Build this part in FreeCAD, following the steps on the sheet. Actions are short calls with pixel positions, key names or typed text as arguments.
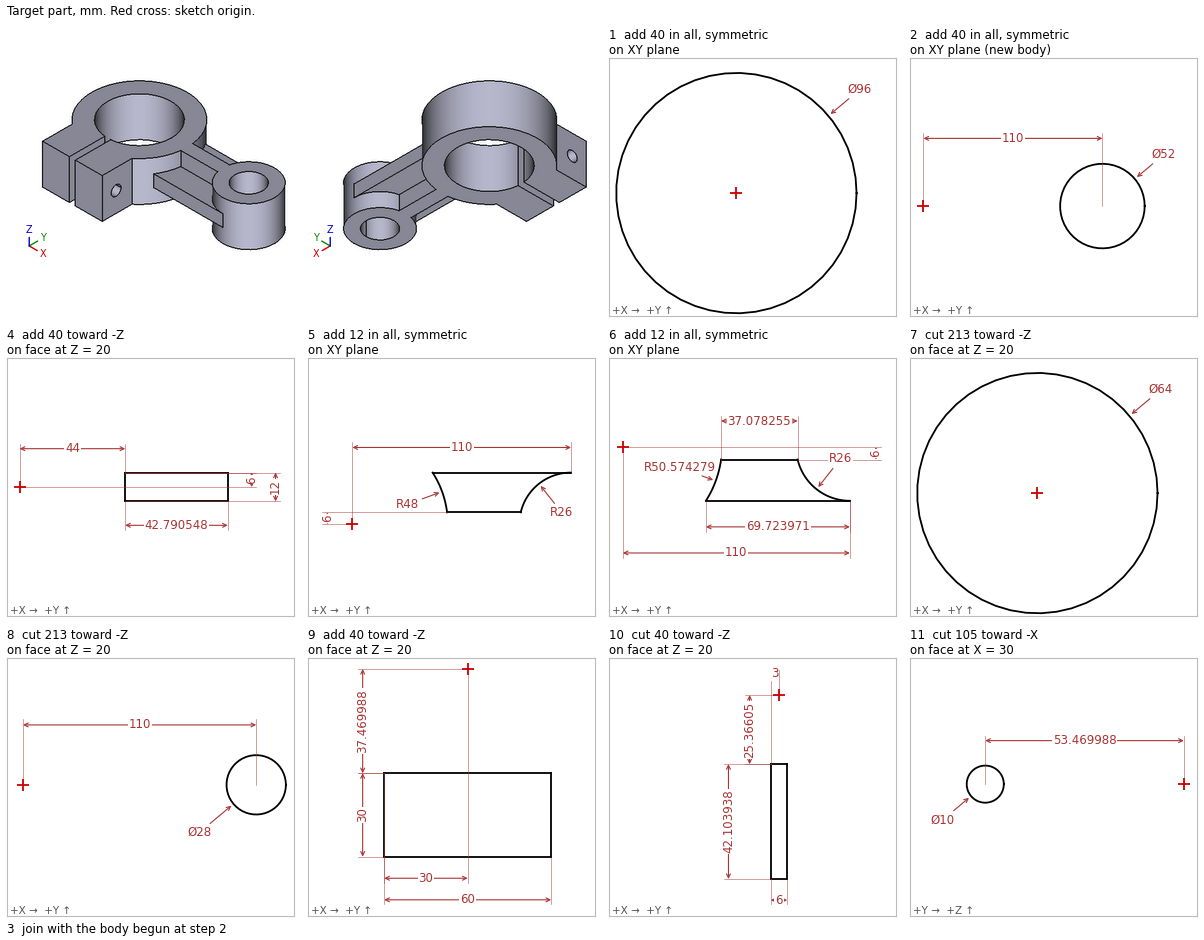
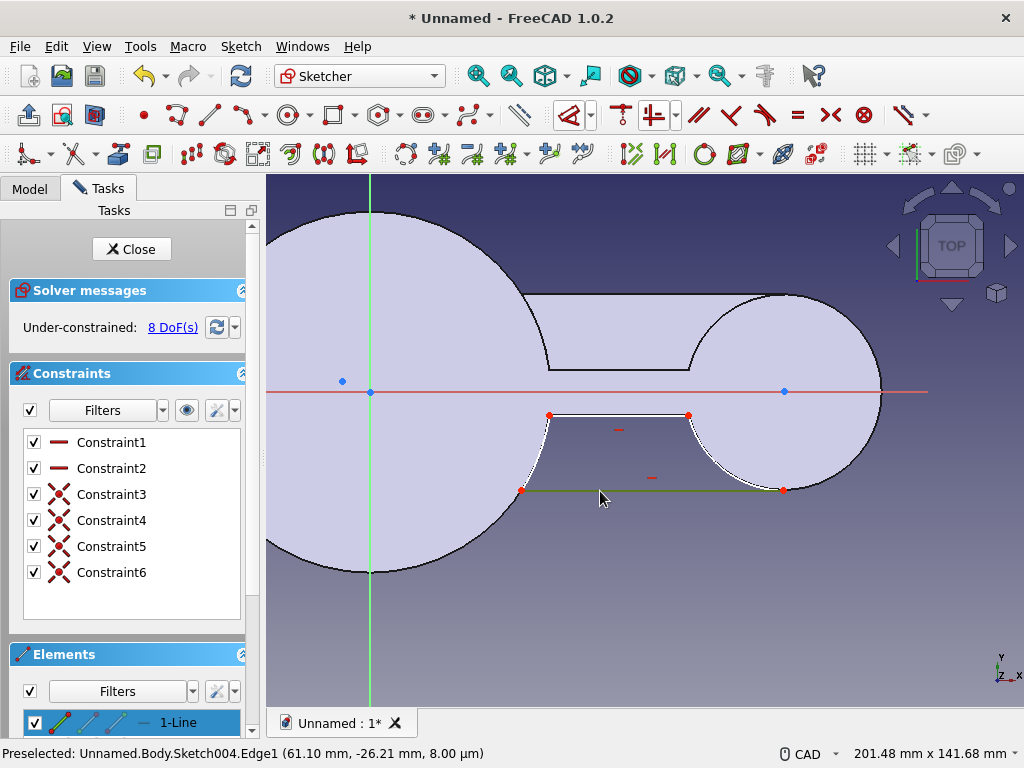
click(705, 451)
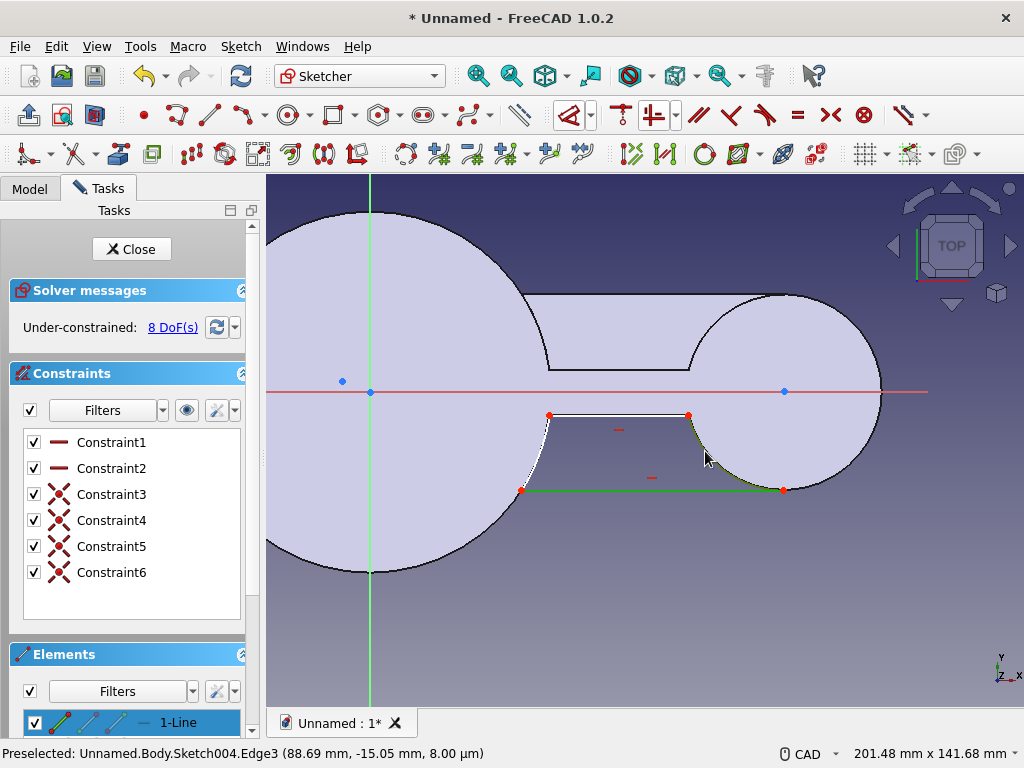
click(765, 116)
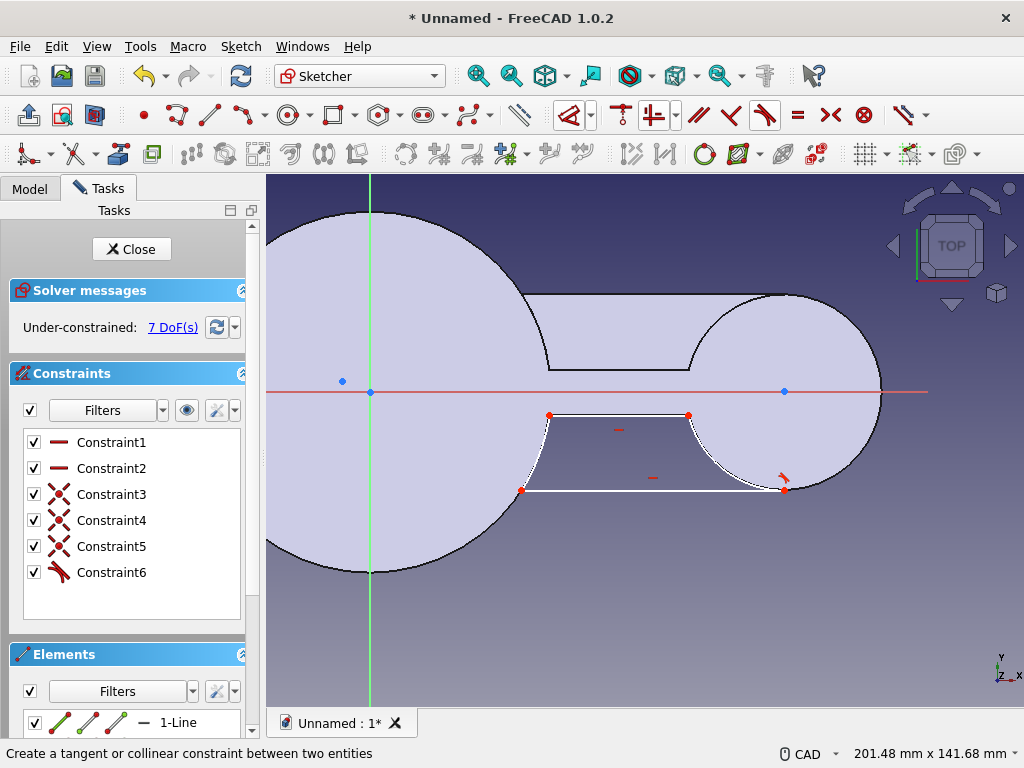
click(785, 392)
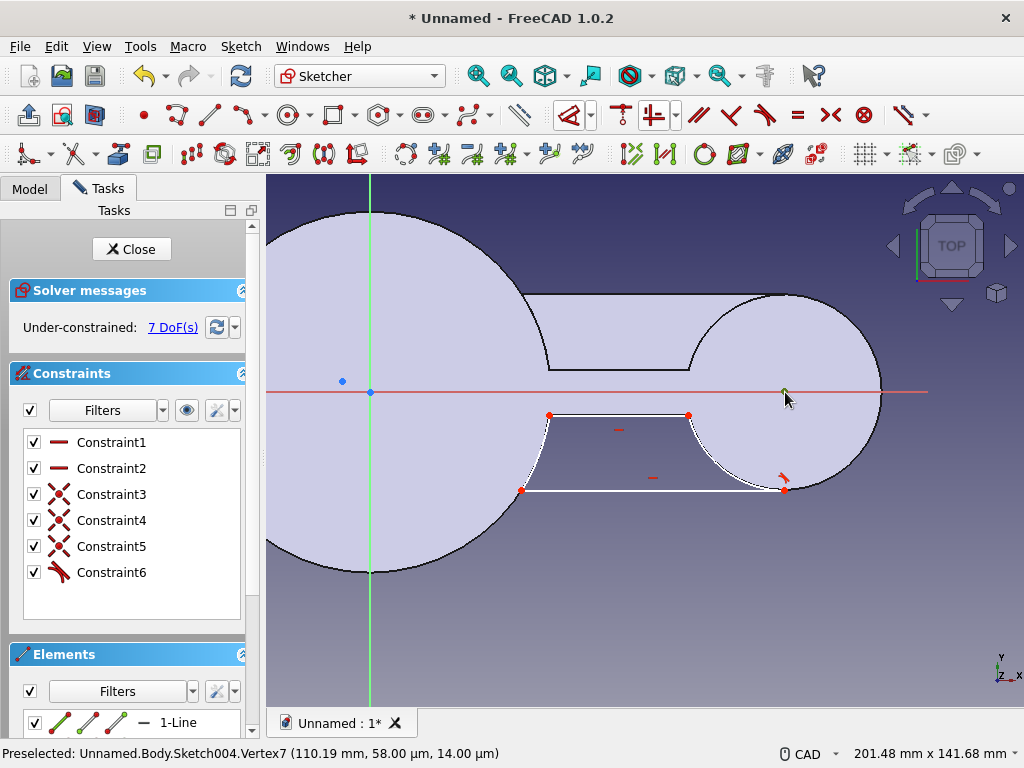
click(334, 392)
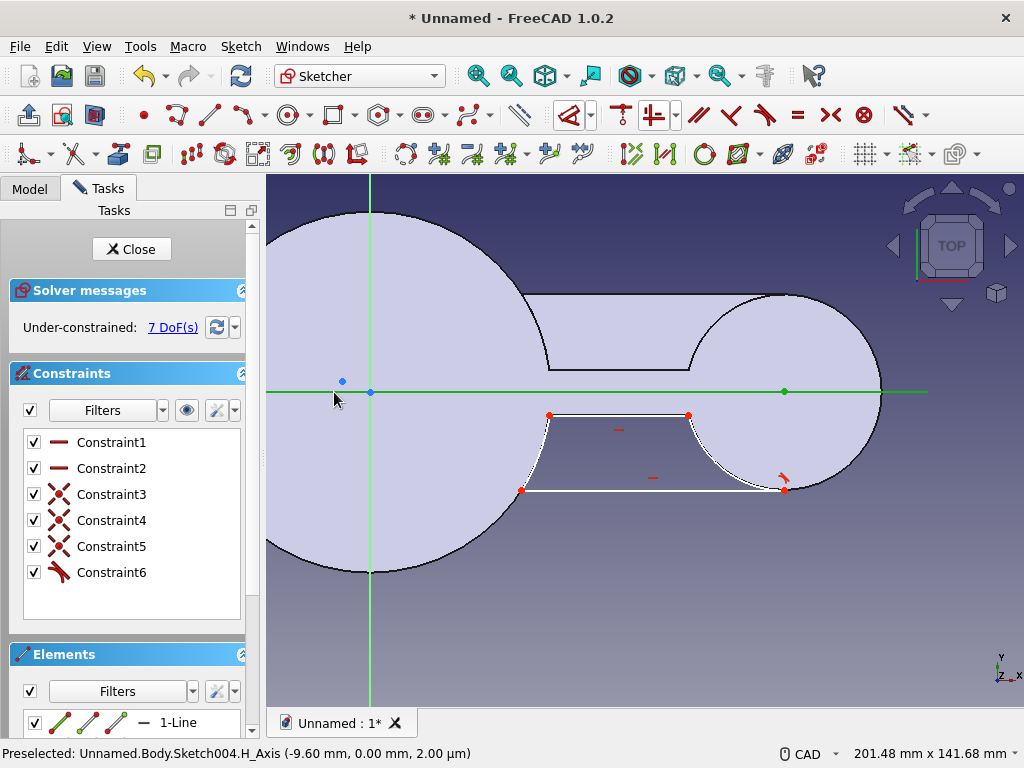
click(621, 116)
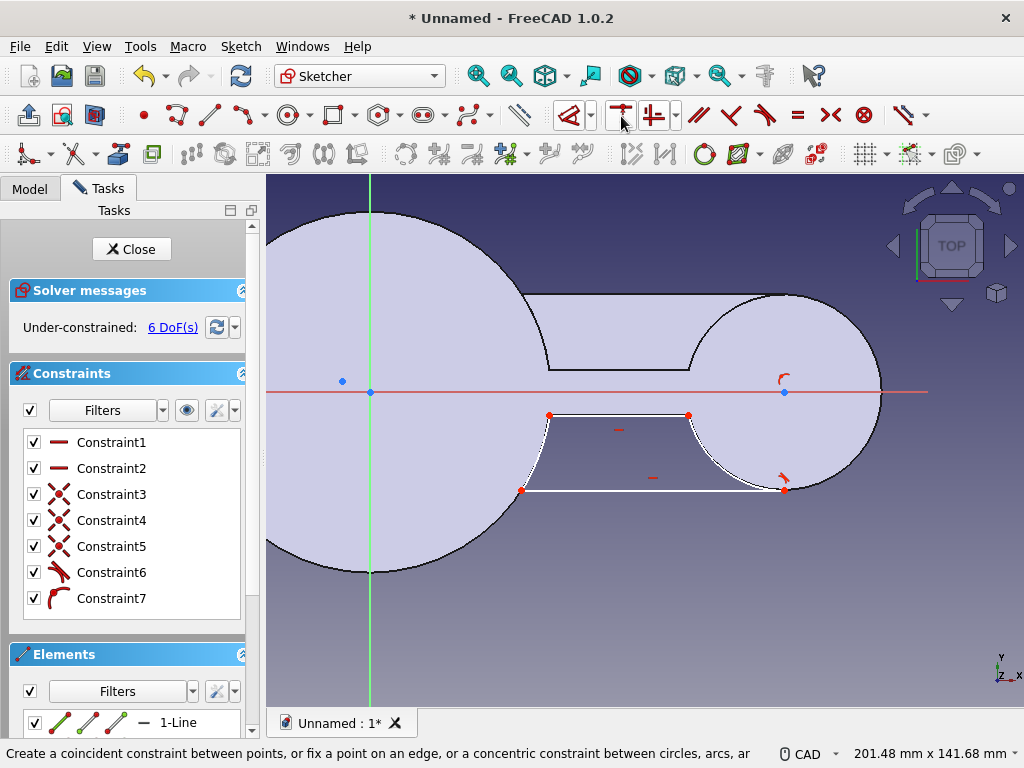
click(705, 451)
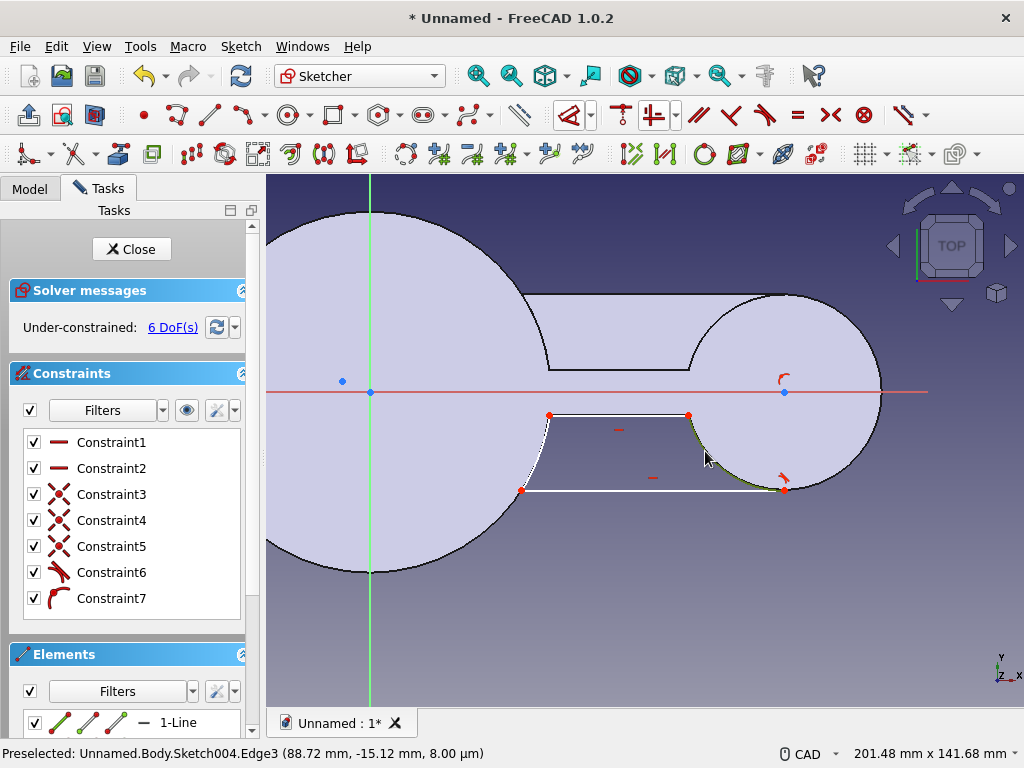
click(590, 116)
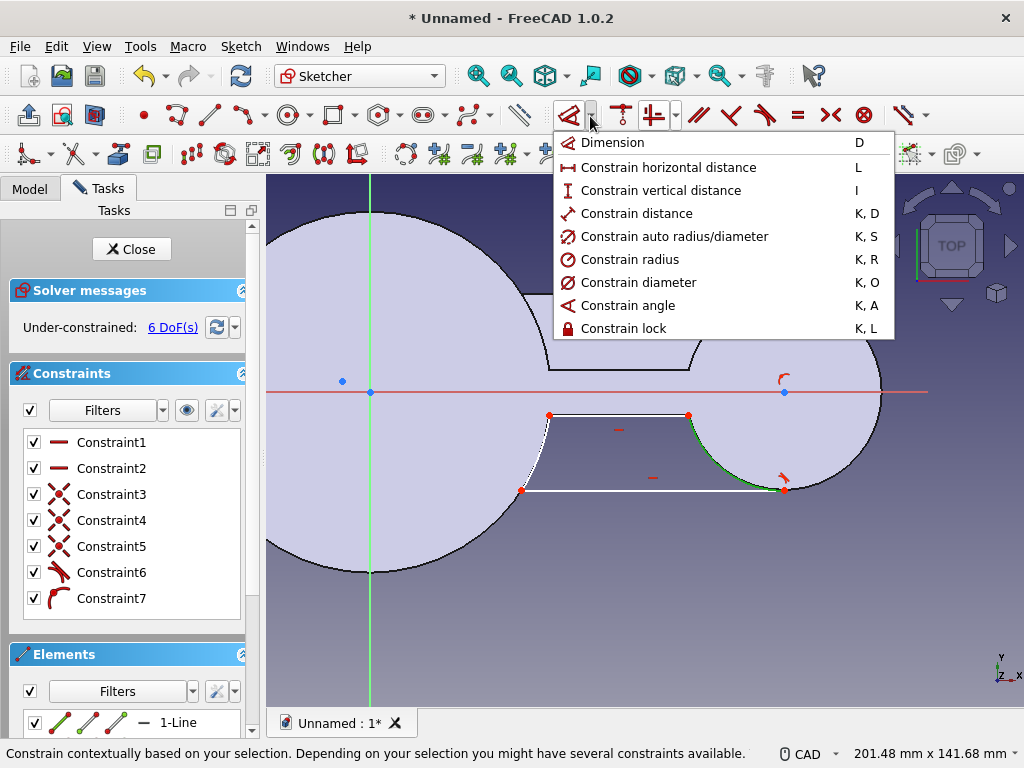
click(724, 260)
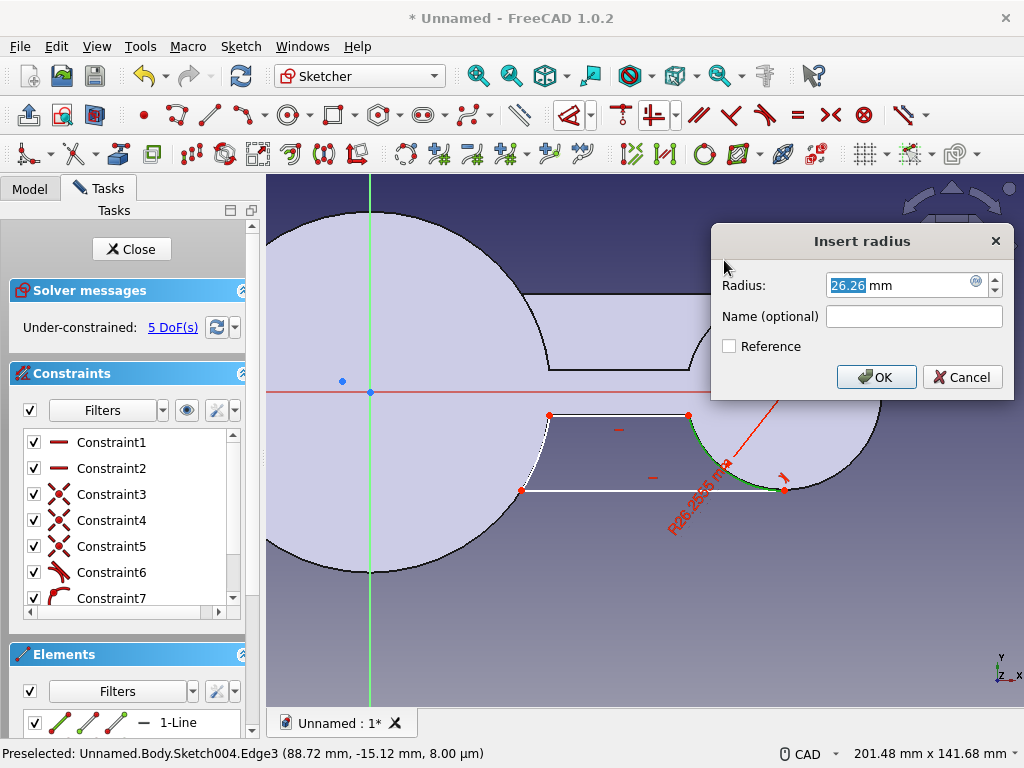
text(26)
key(Return)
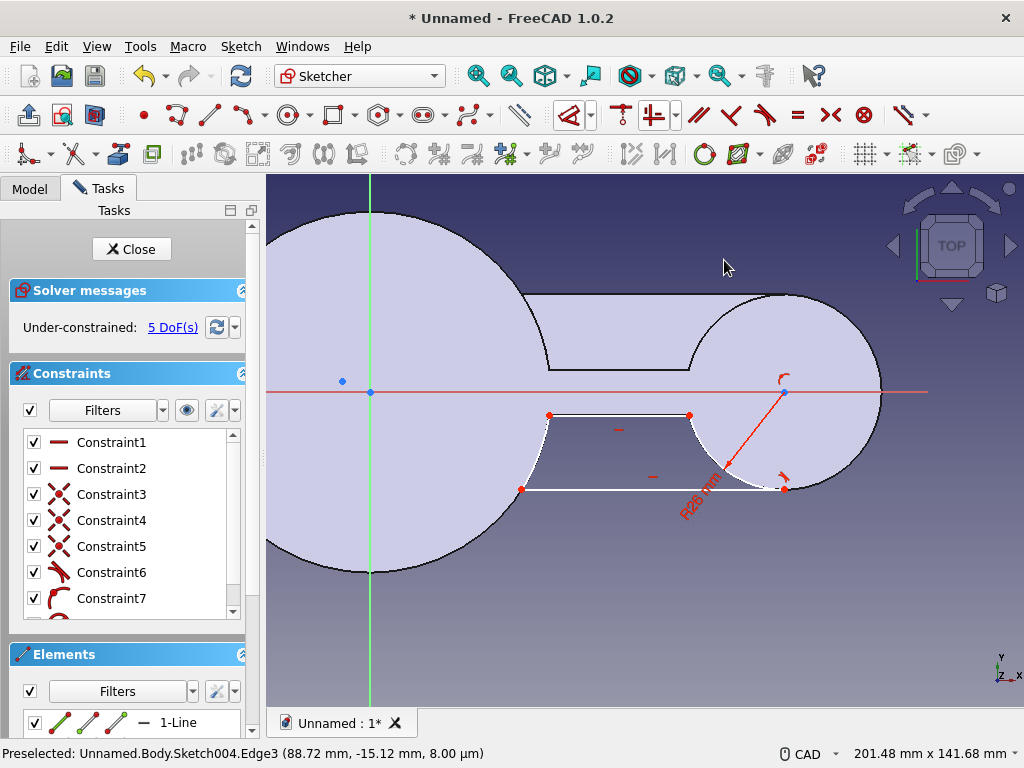
click(533, 469)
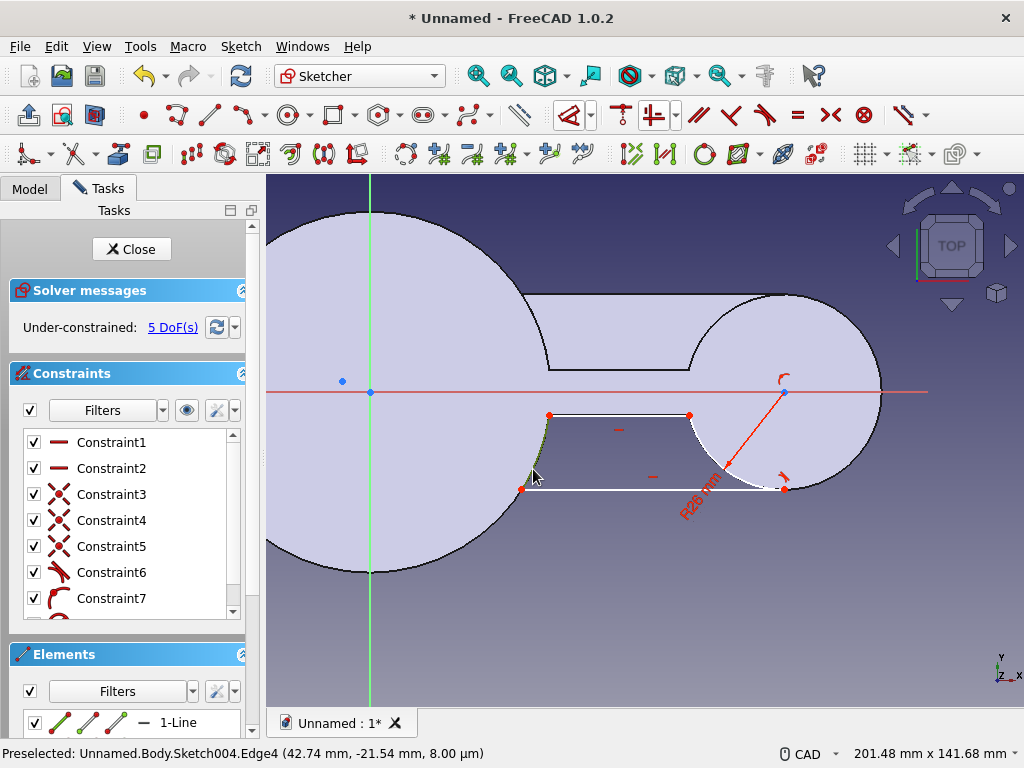
key(k)
key(r)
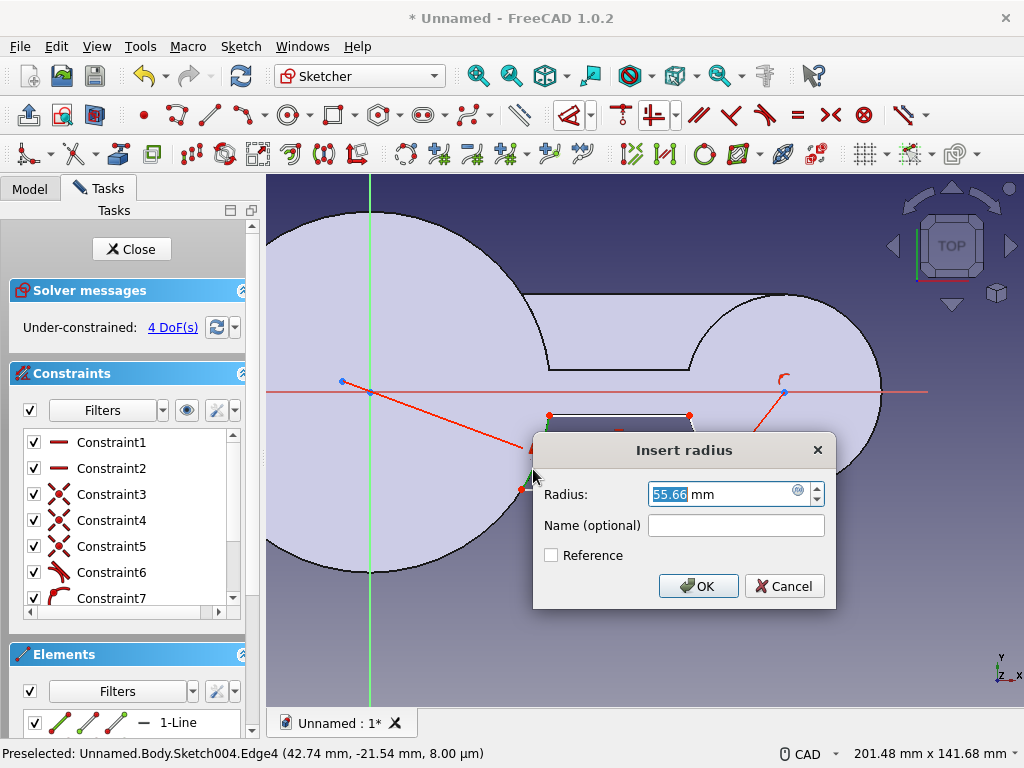
text(50.574279)
key(Return)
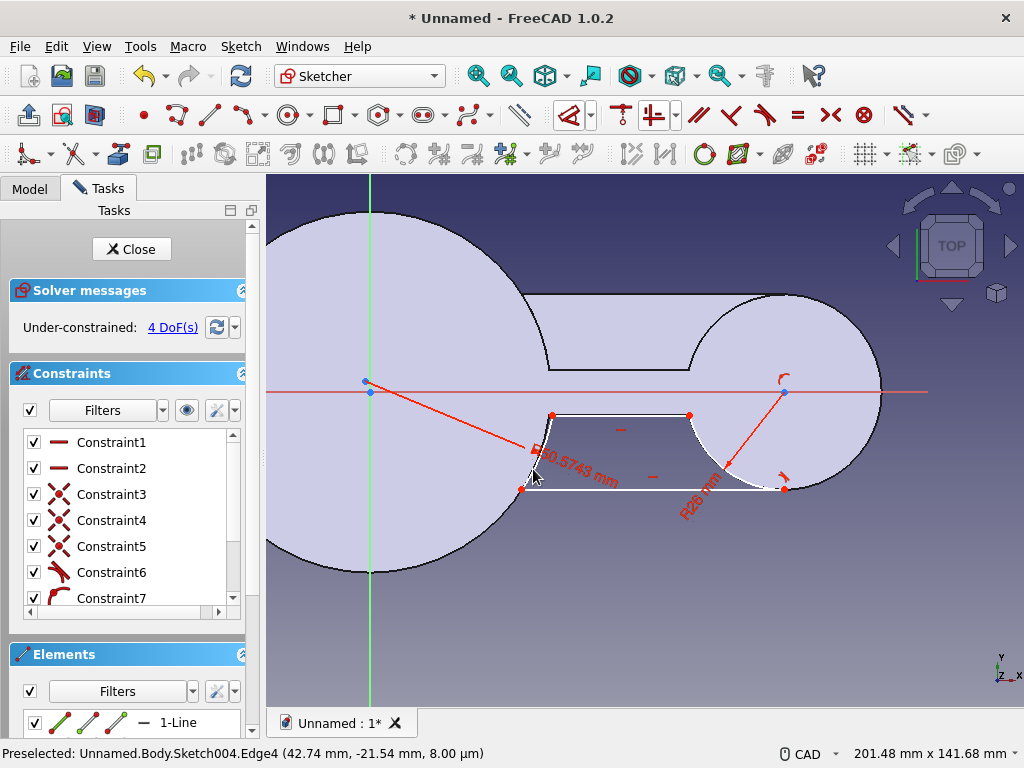
scroll(690, 416, up, 3)